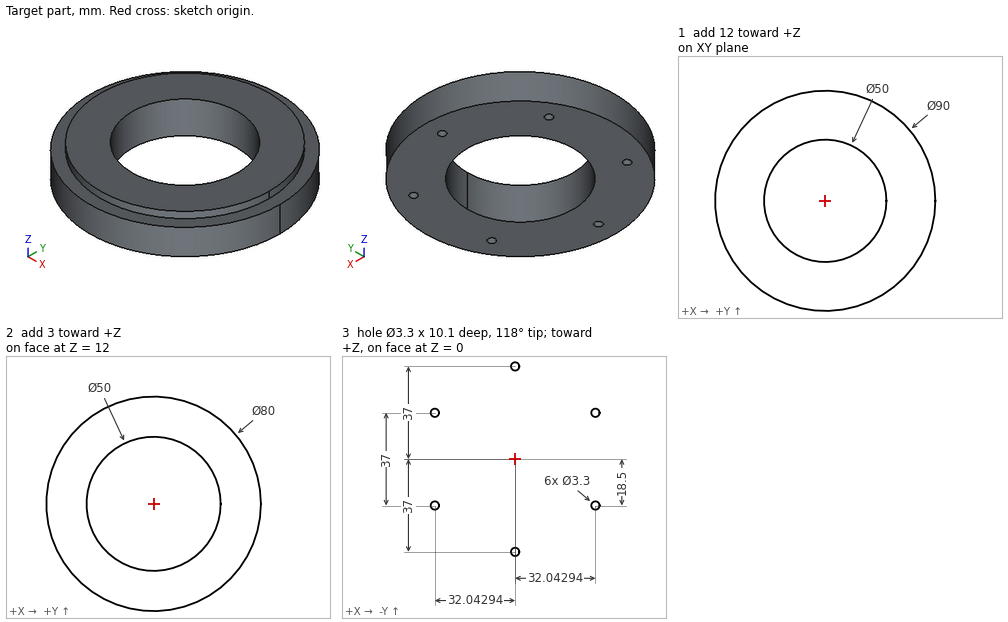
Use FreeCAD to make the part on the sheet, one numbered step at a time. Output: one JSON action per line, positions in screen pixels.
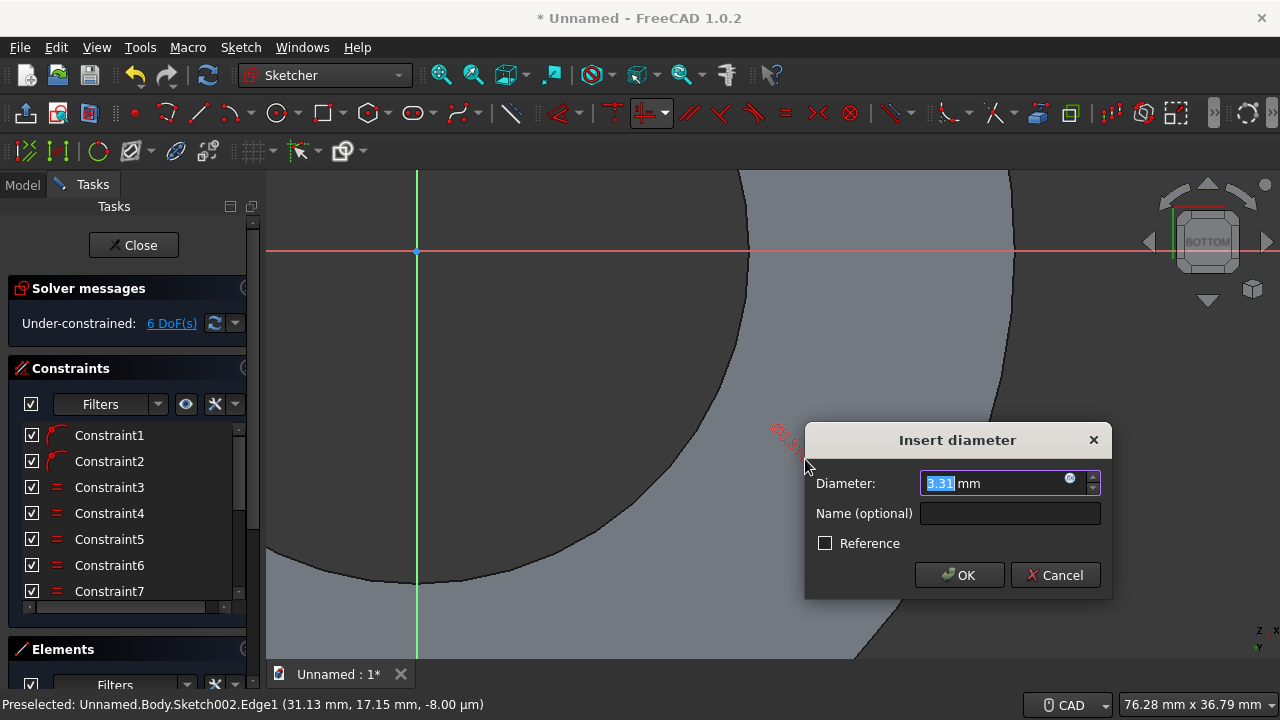
{"action": "type", "text": "3.3"}
{"action": "key", "text": "Return"}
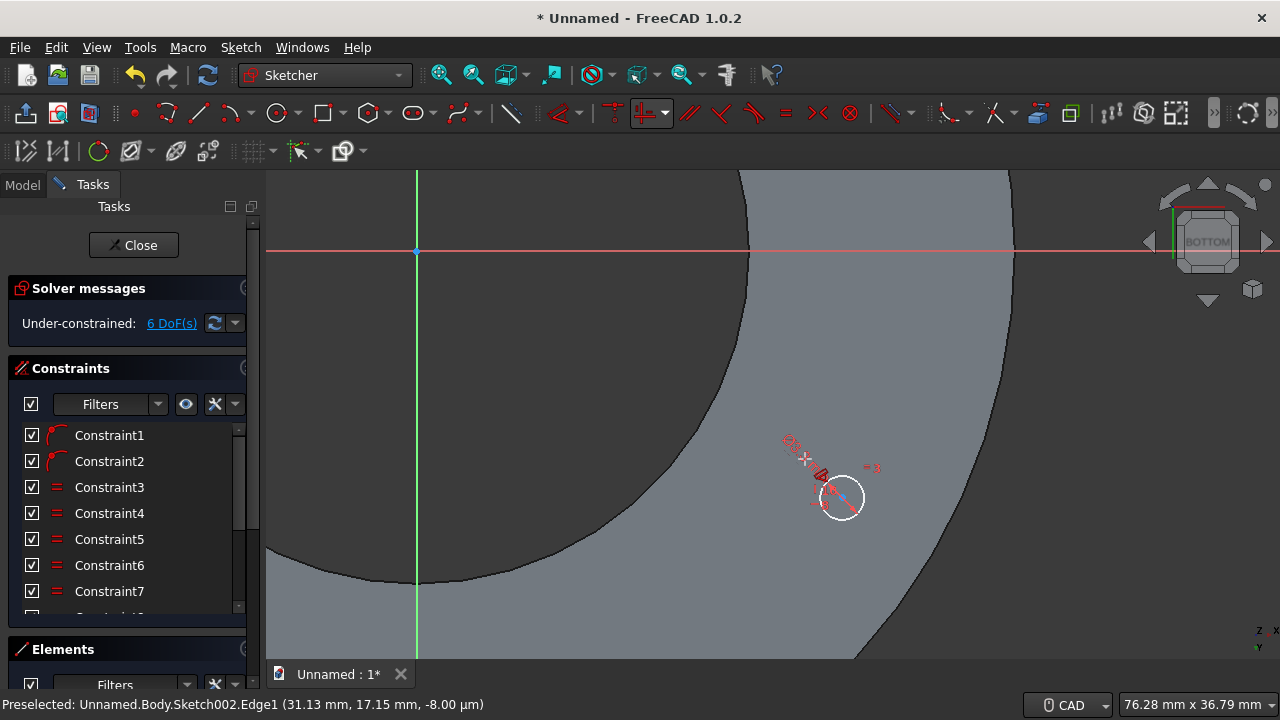
{"action": "scroll", "coordinate": [829, 485], "scroll_direction": "down", "scroll_amount": 6}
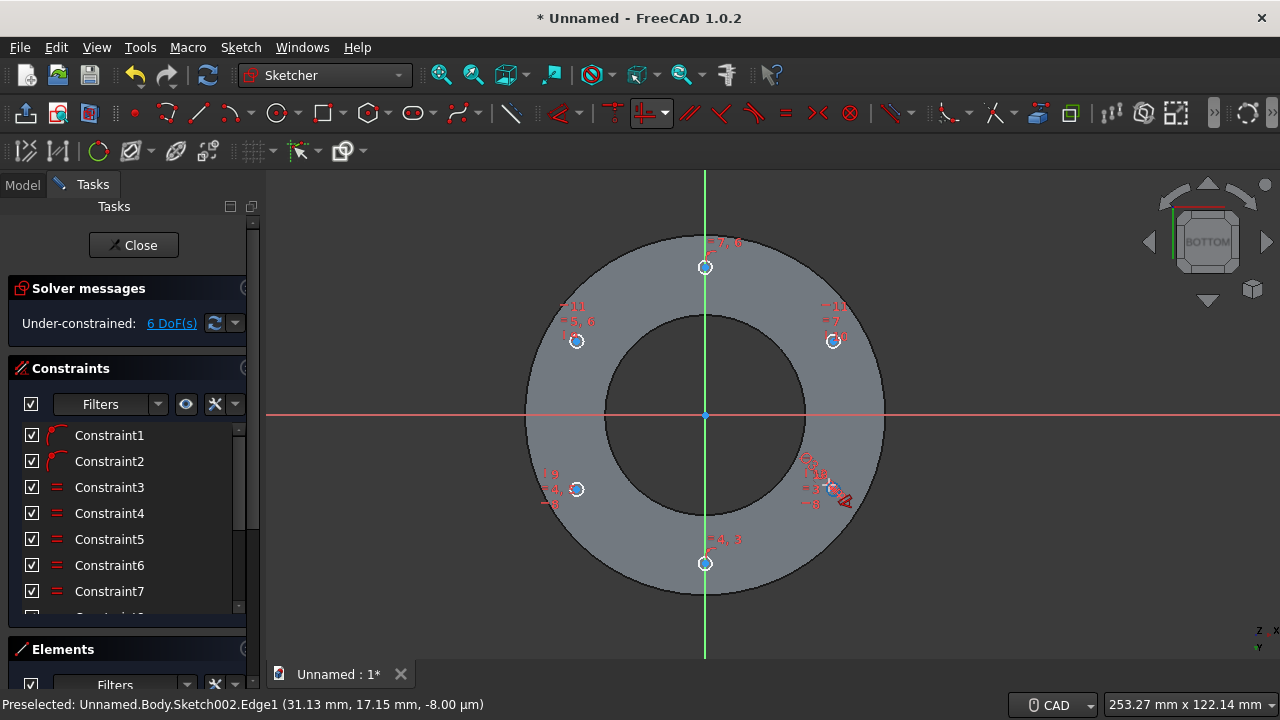
{"action": "left_click", "coordinate": [705, 564]}
{"action": "left_click", "coordinate": [739, 489]}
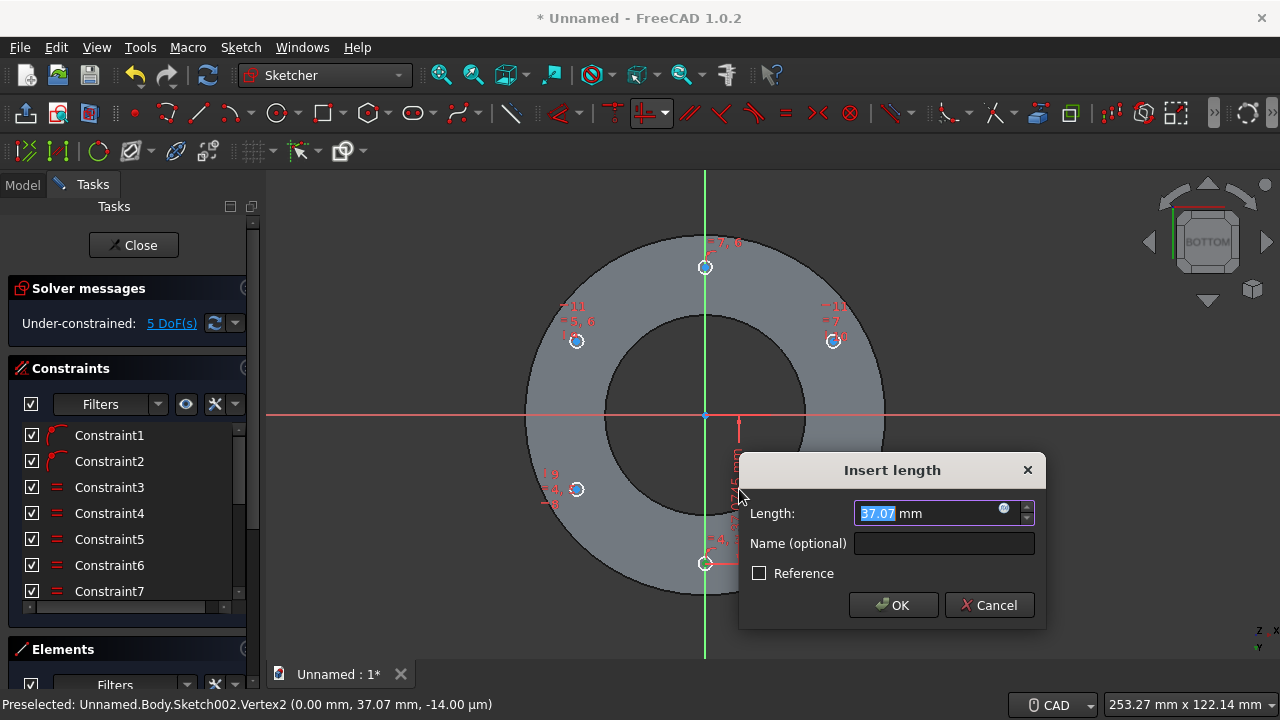
{"action": "type", "text": "37"}
{"action": "key", "text": "Return"}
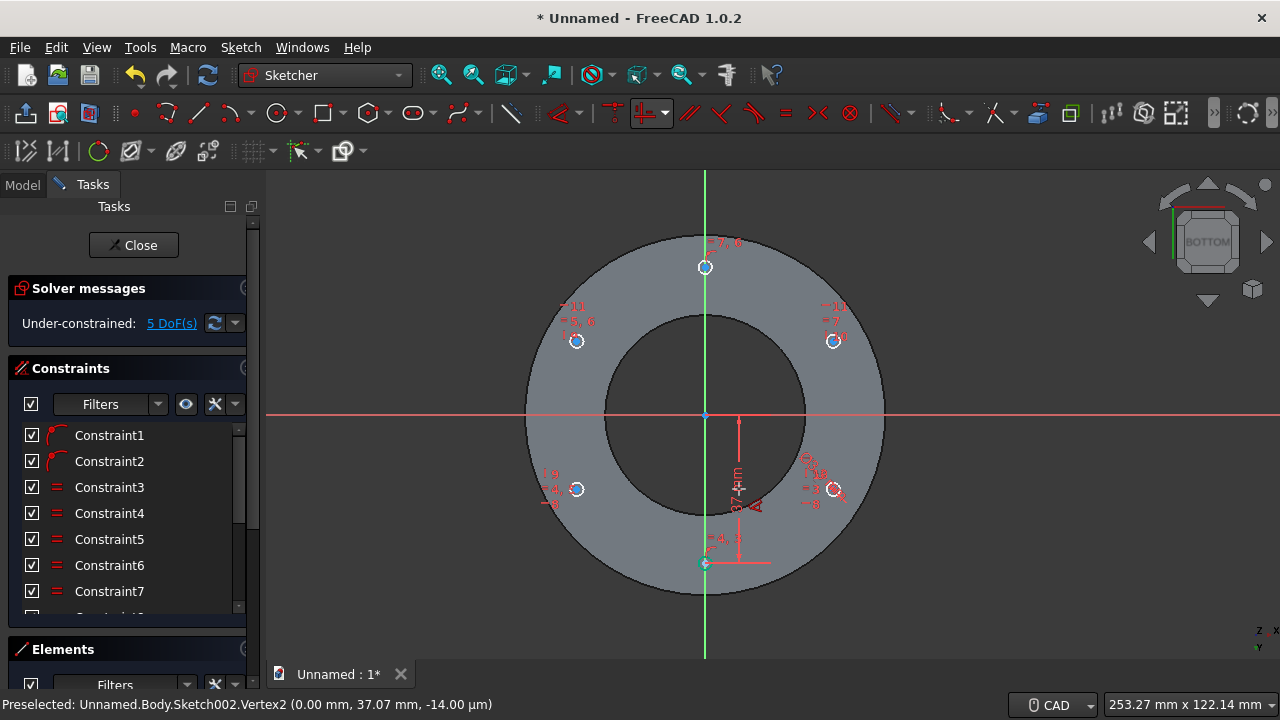
{"action": "left_click", "coordinate": [705, 267]}
{"action": "left_click", "coordinate": [739, 341]}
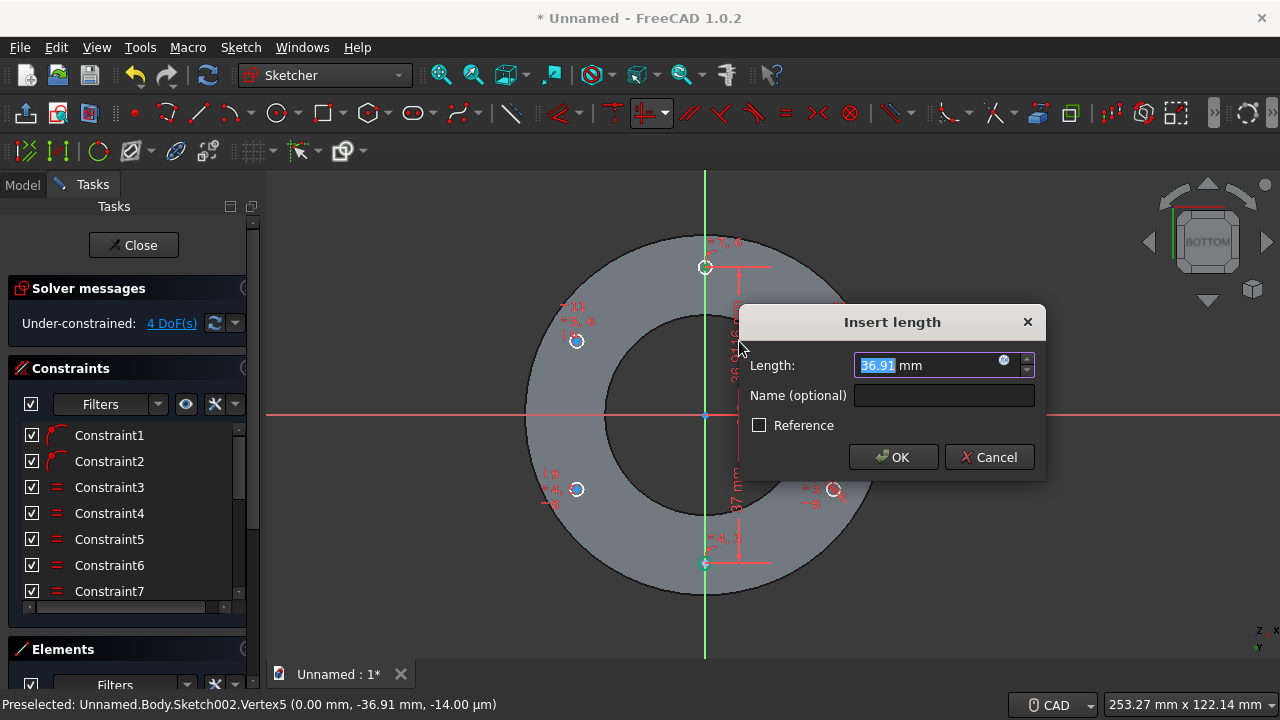
{"action": "type", "text": "37"}
{"action": "key", "text": "Return"}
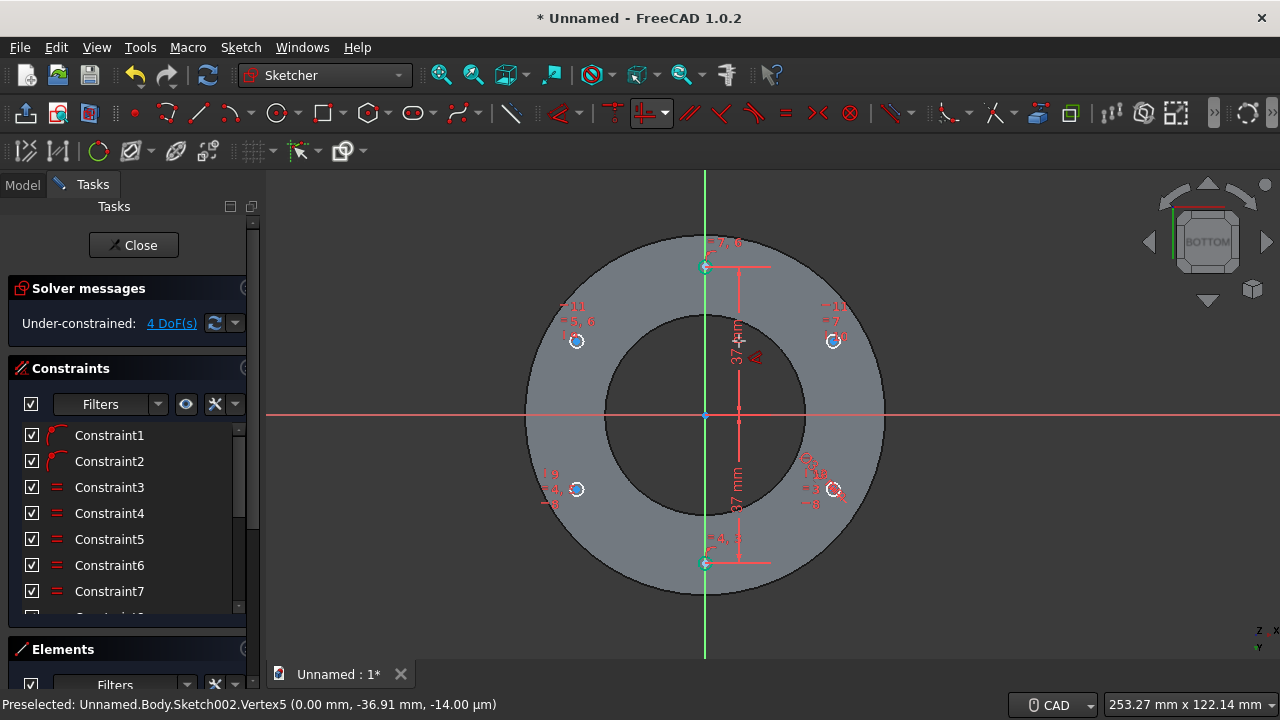
{"action": "left_click", "coordinate": [577, 489]}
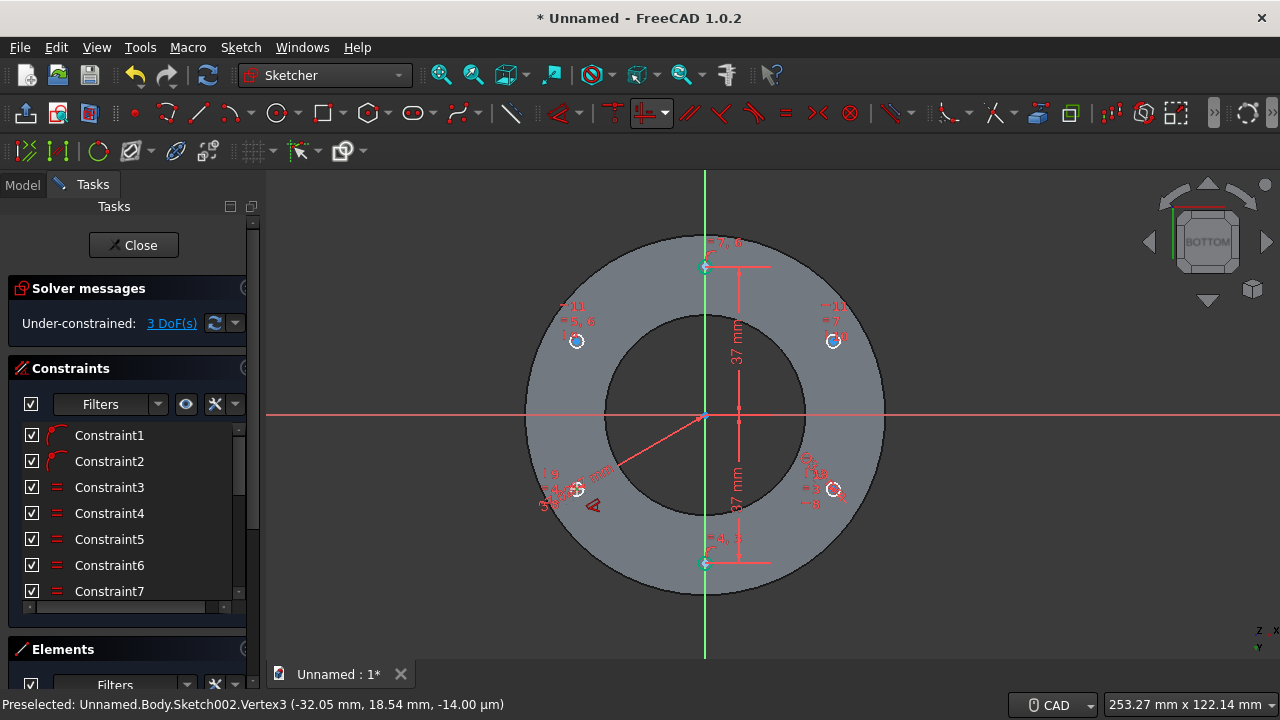
{"action": "left_click", "coordinate": [577, 341]}
{"action": "left_click", "coordinate": [543, 381]}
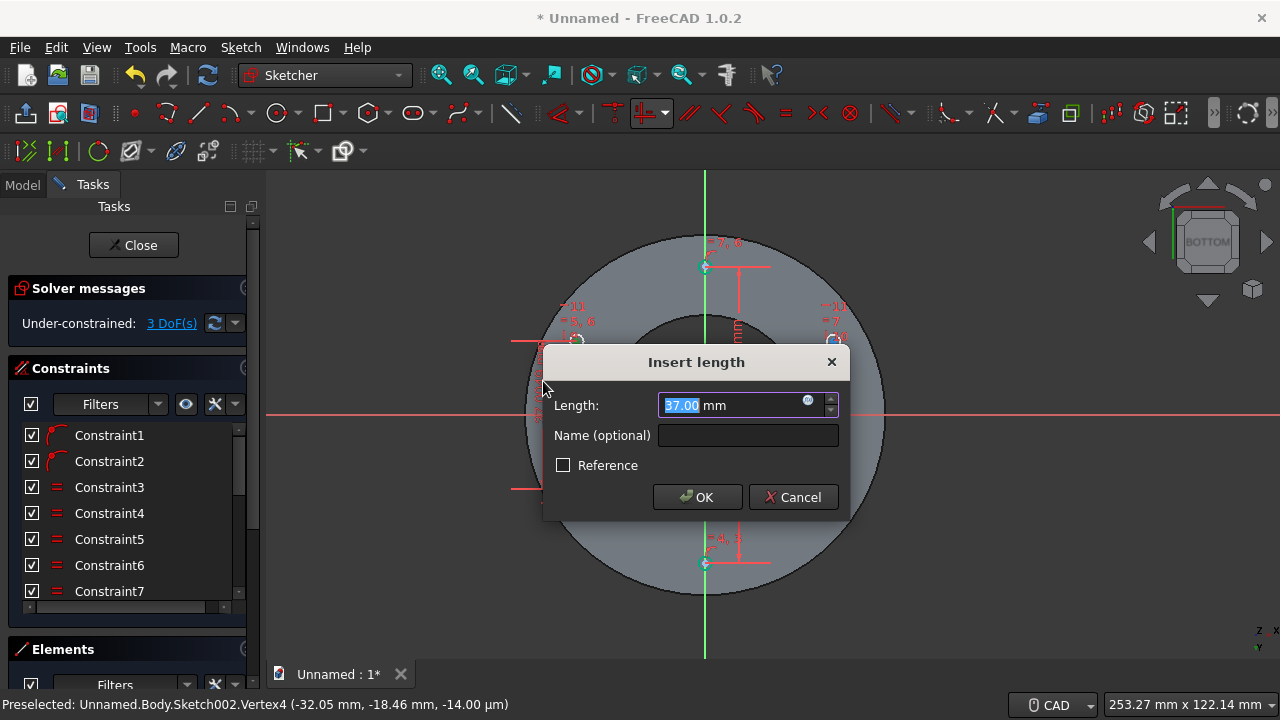
{"action": "type", "text": "37"}
{"action": "key", "text": "Return"}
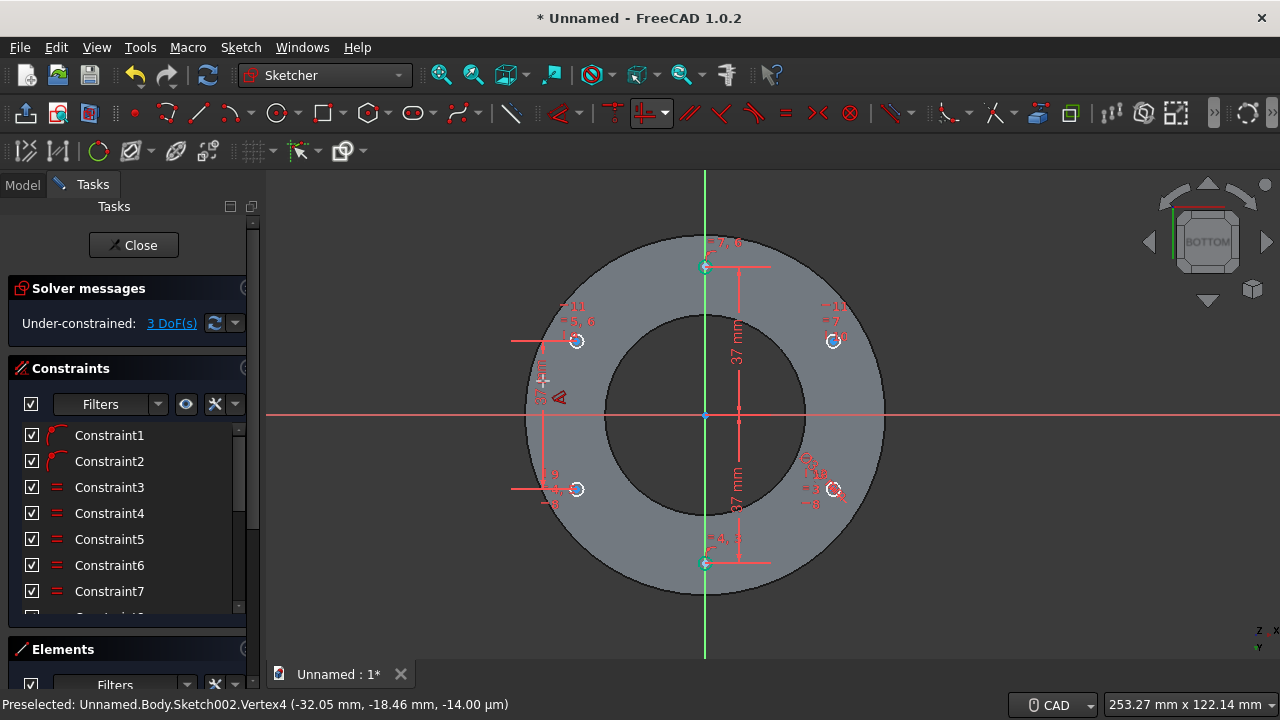
{"action": "left_click", "coordinate": [833, 489]}
{"action": "left_click", "coordinate": [867, 452]}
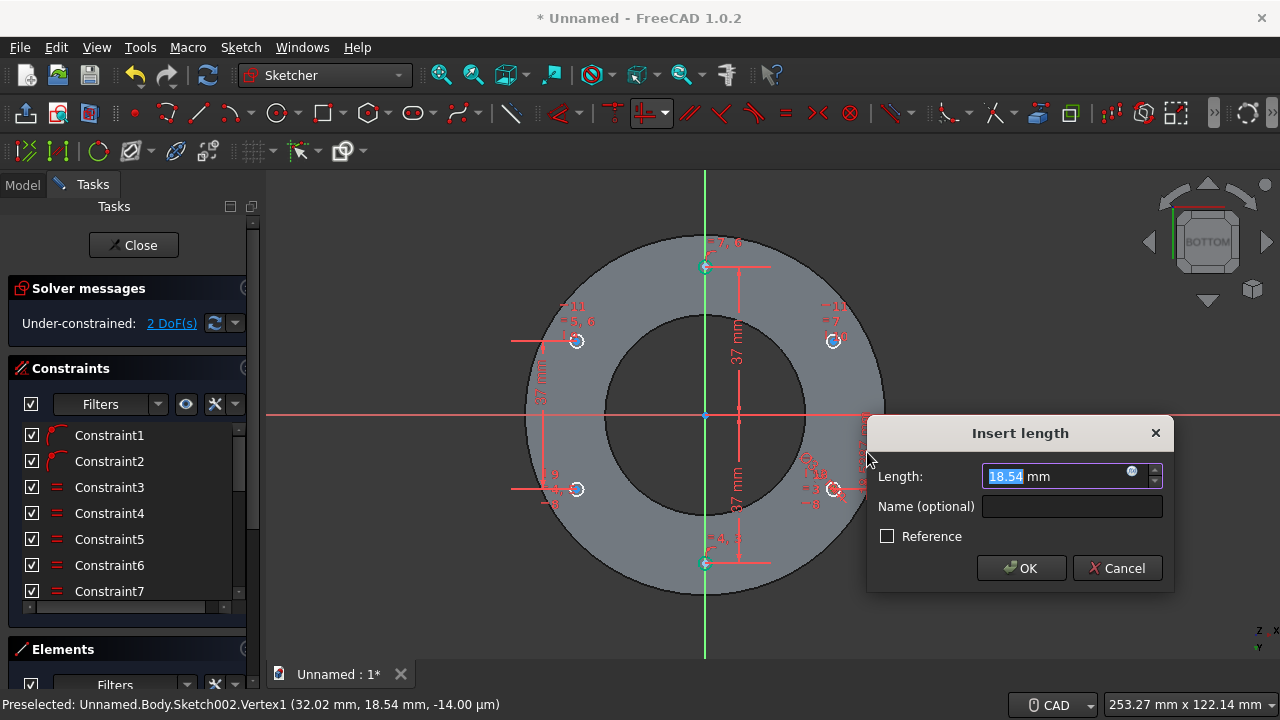
{"action": "type", "text": "18.5"}
{"action": "key", "text": "Return"}